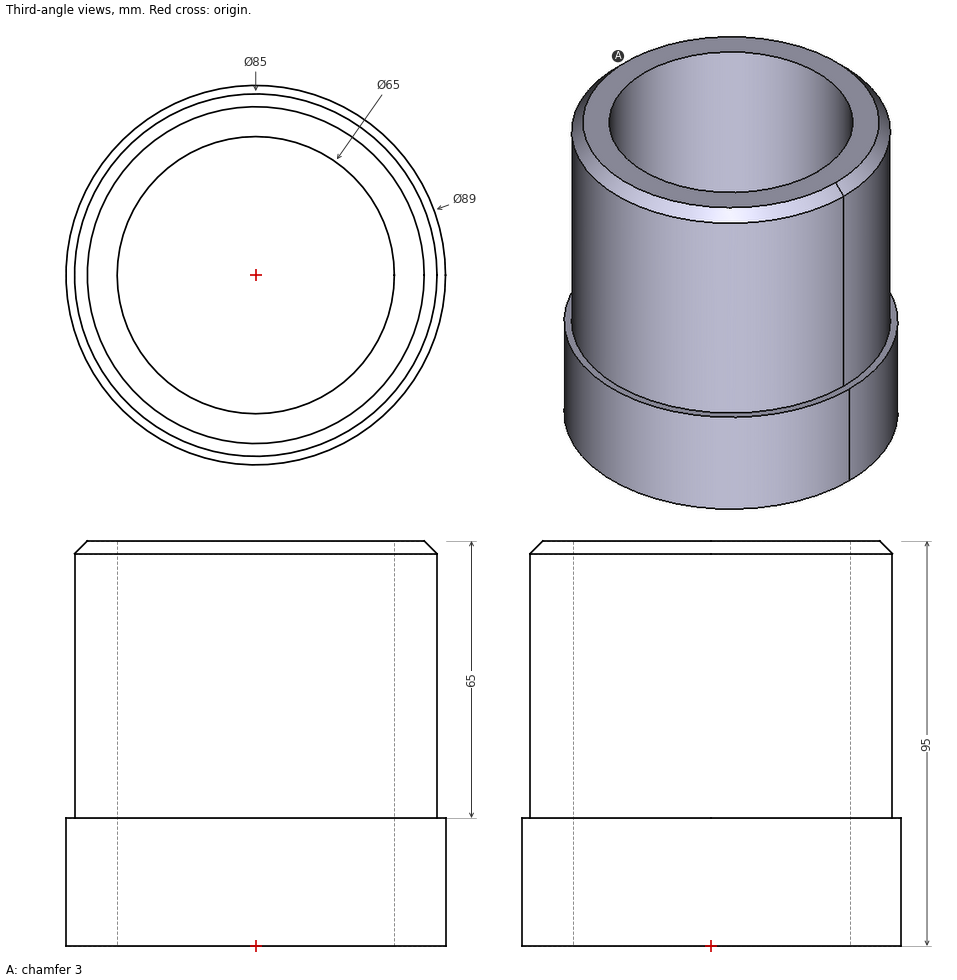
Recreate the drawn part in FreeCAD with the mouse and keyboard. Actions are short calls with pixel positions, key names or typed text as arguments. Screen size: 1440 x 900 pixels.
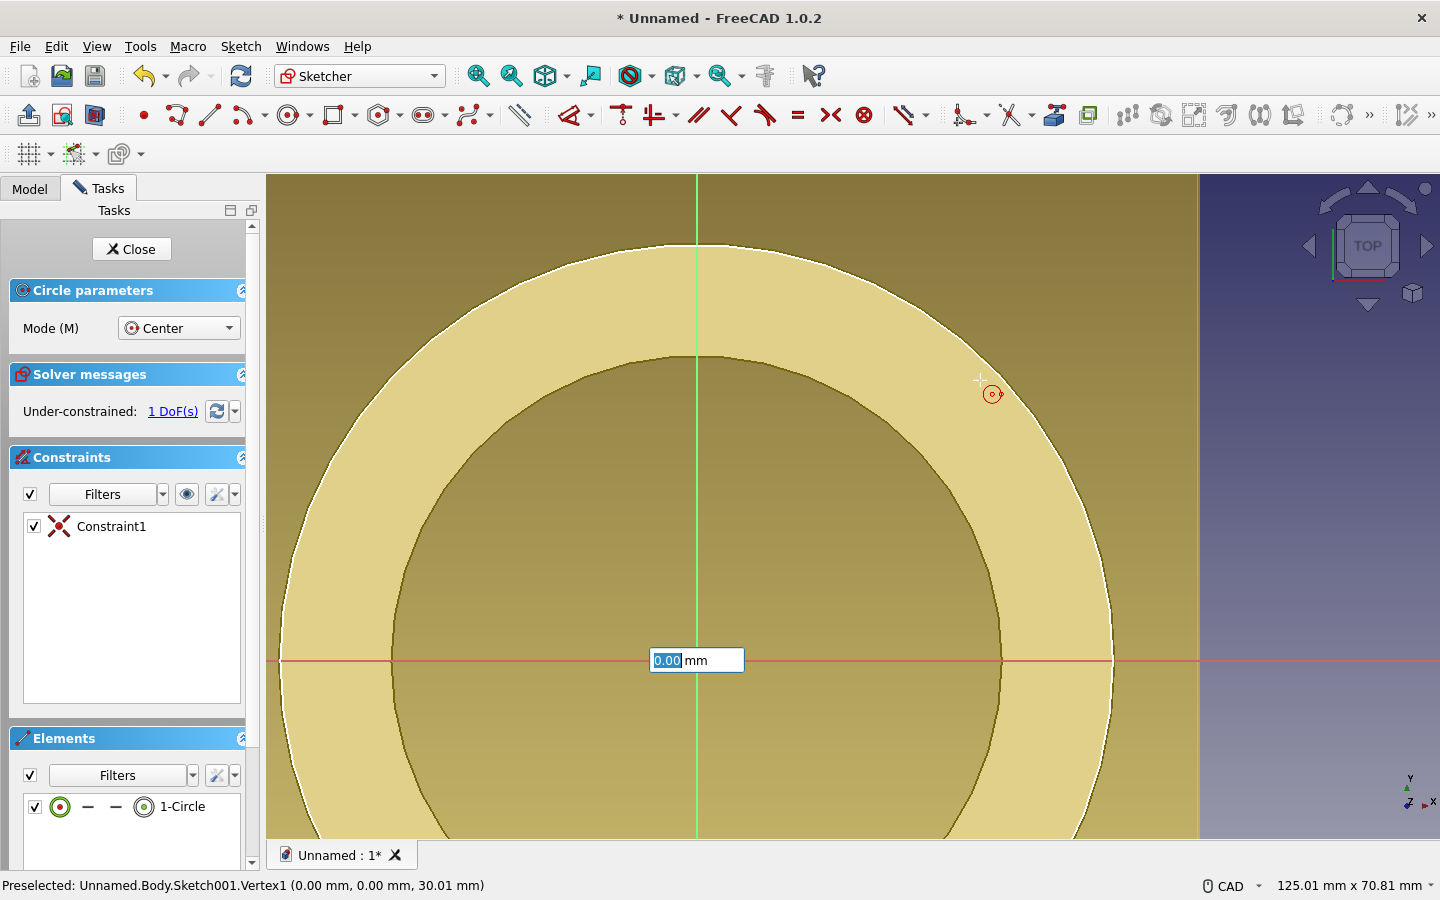
click(979, 379)
key(Escape)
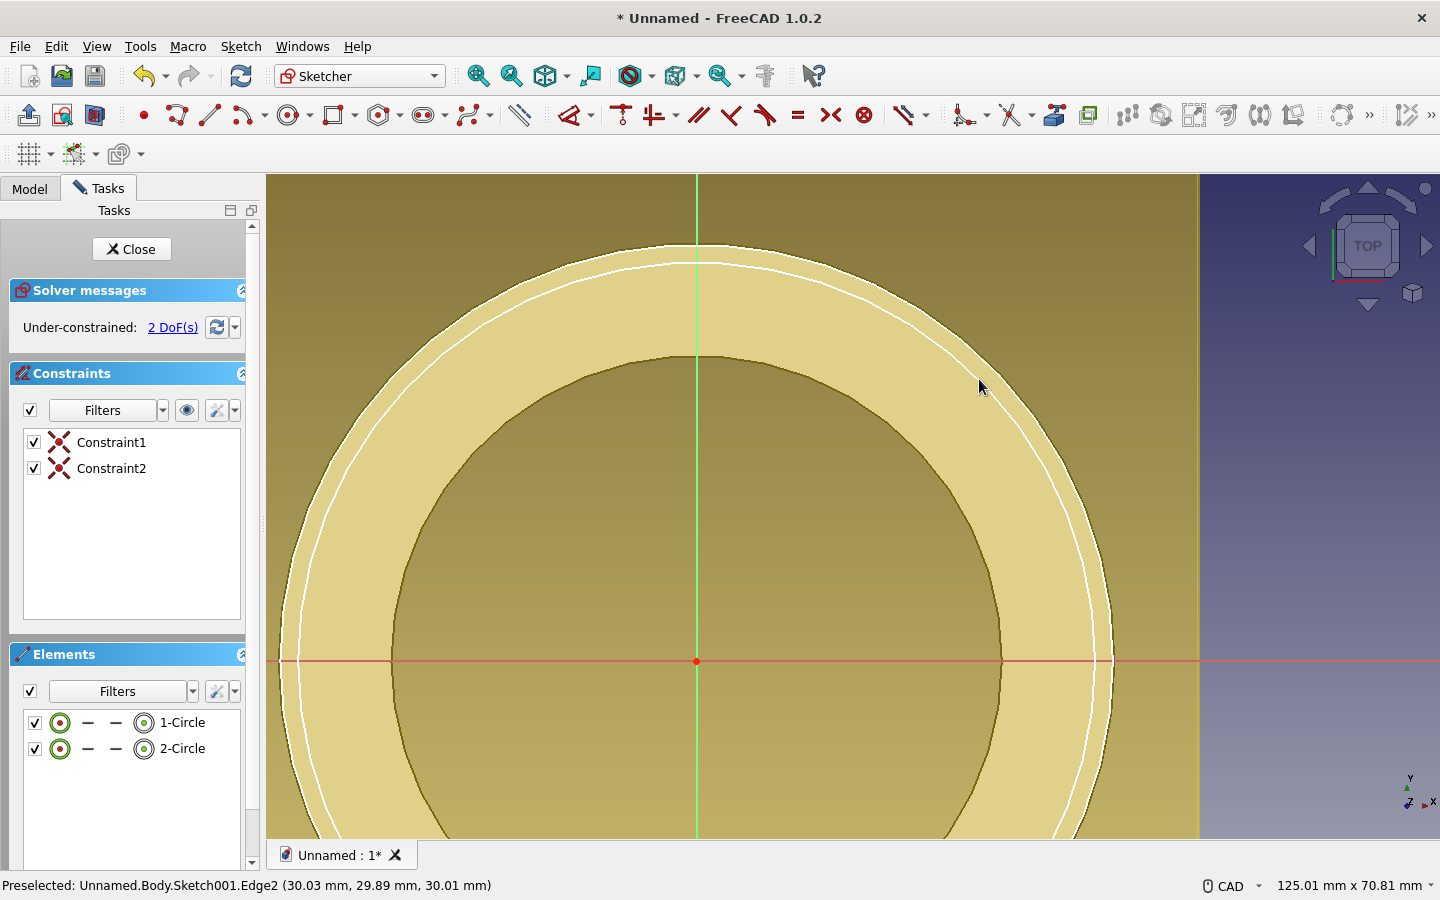
key(d)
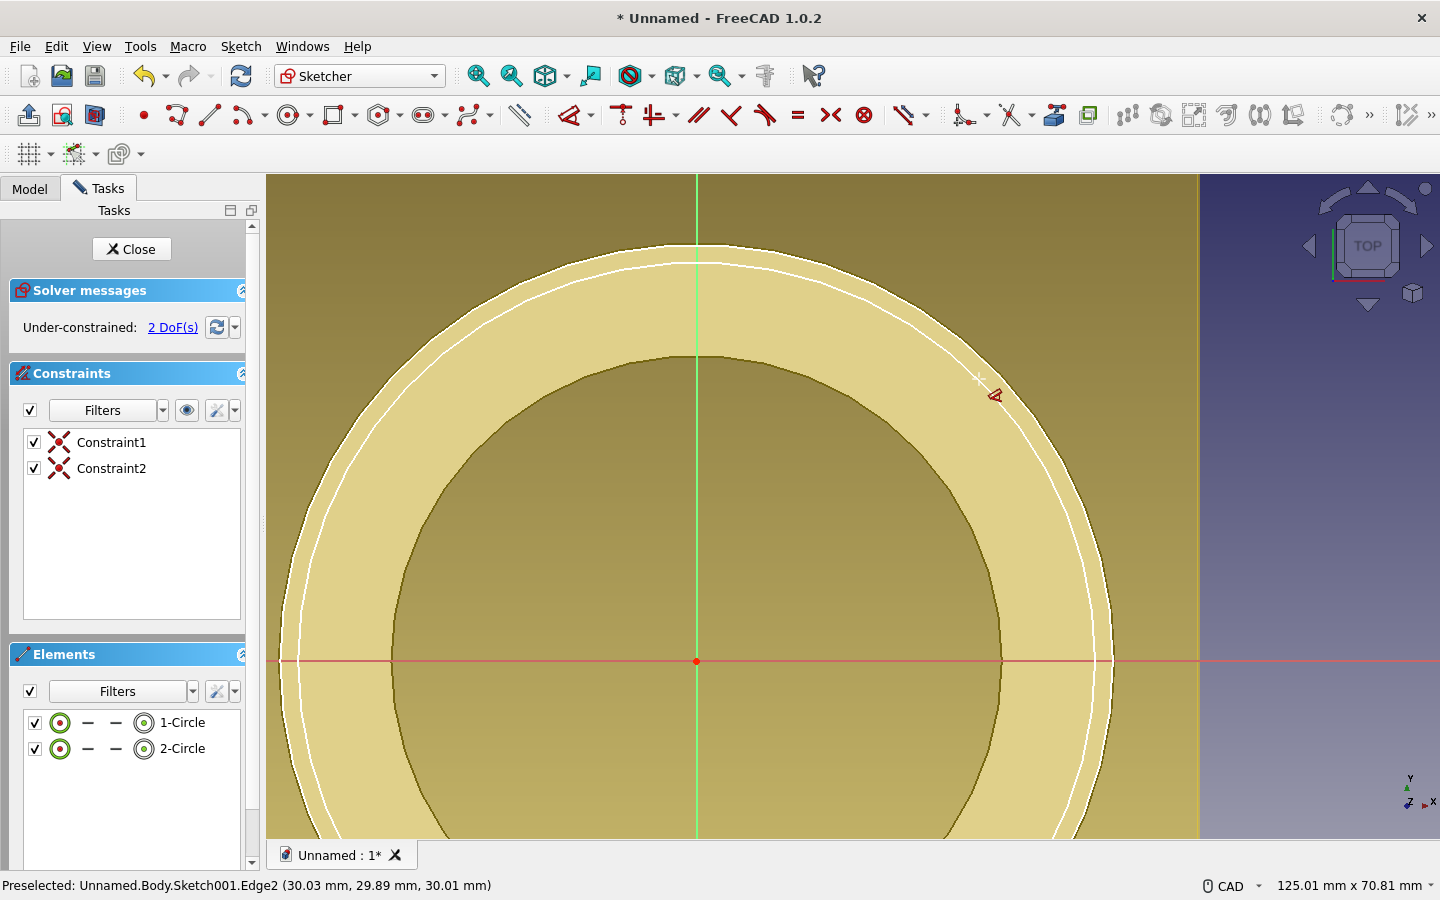
click(990, 366)
click(1013, 343)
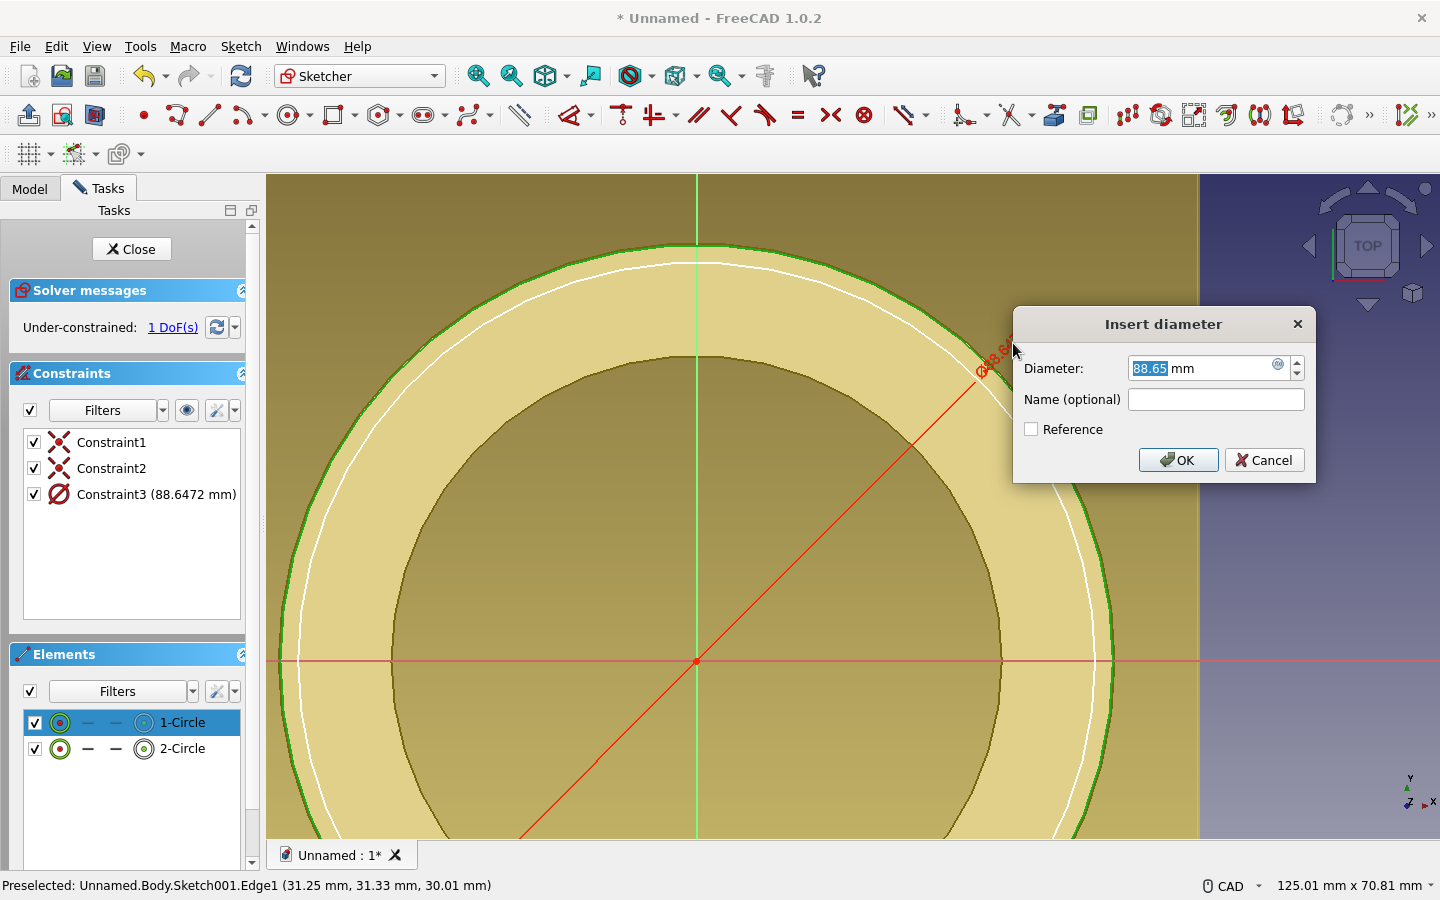
text(89)
key(Return)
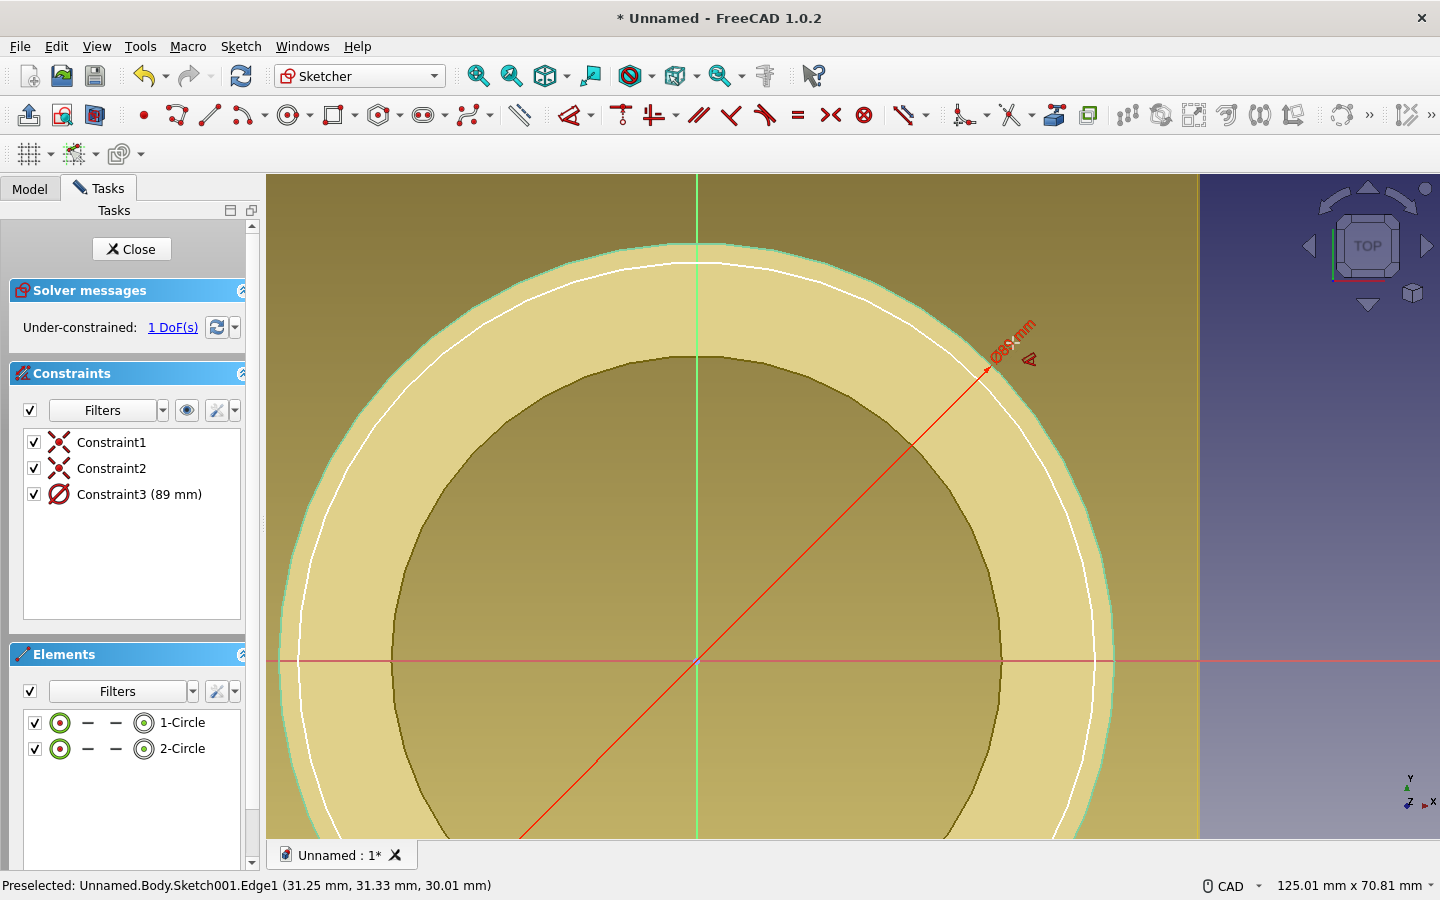
click(978, 379)
click(1132, 533)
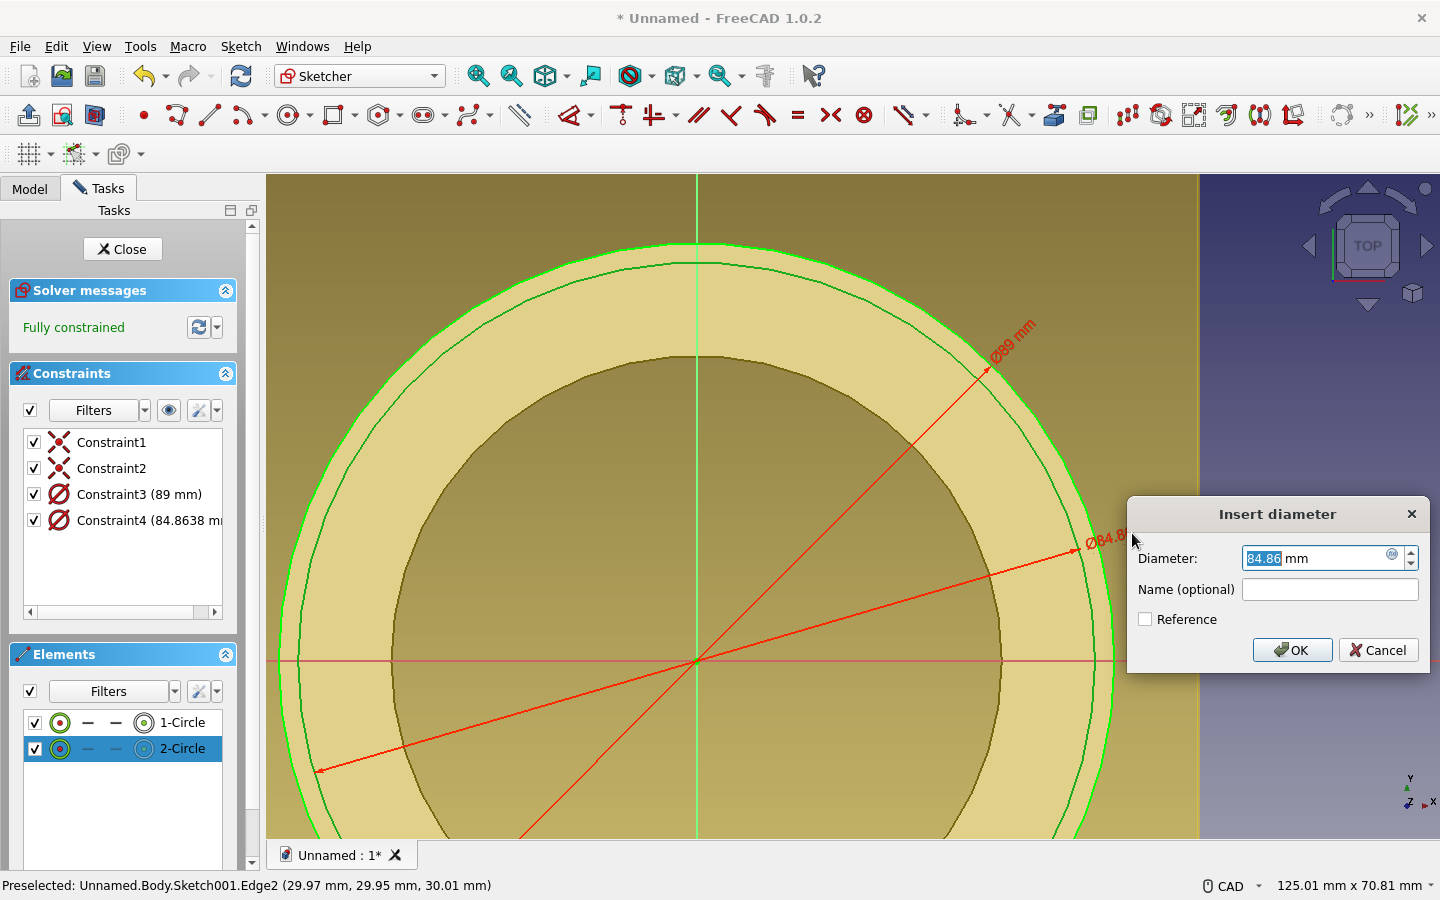
text(85)
key(Return)
key(Escape)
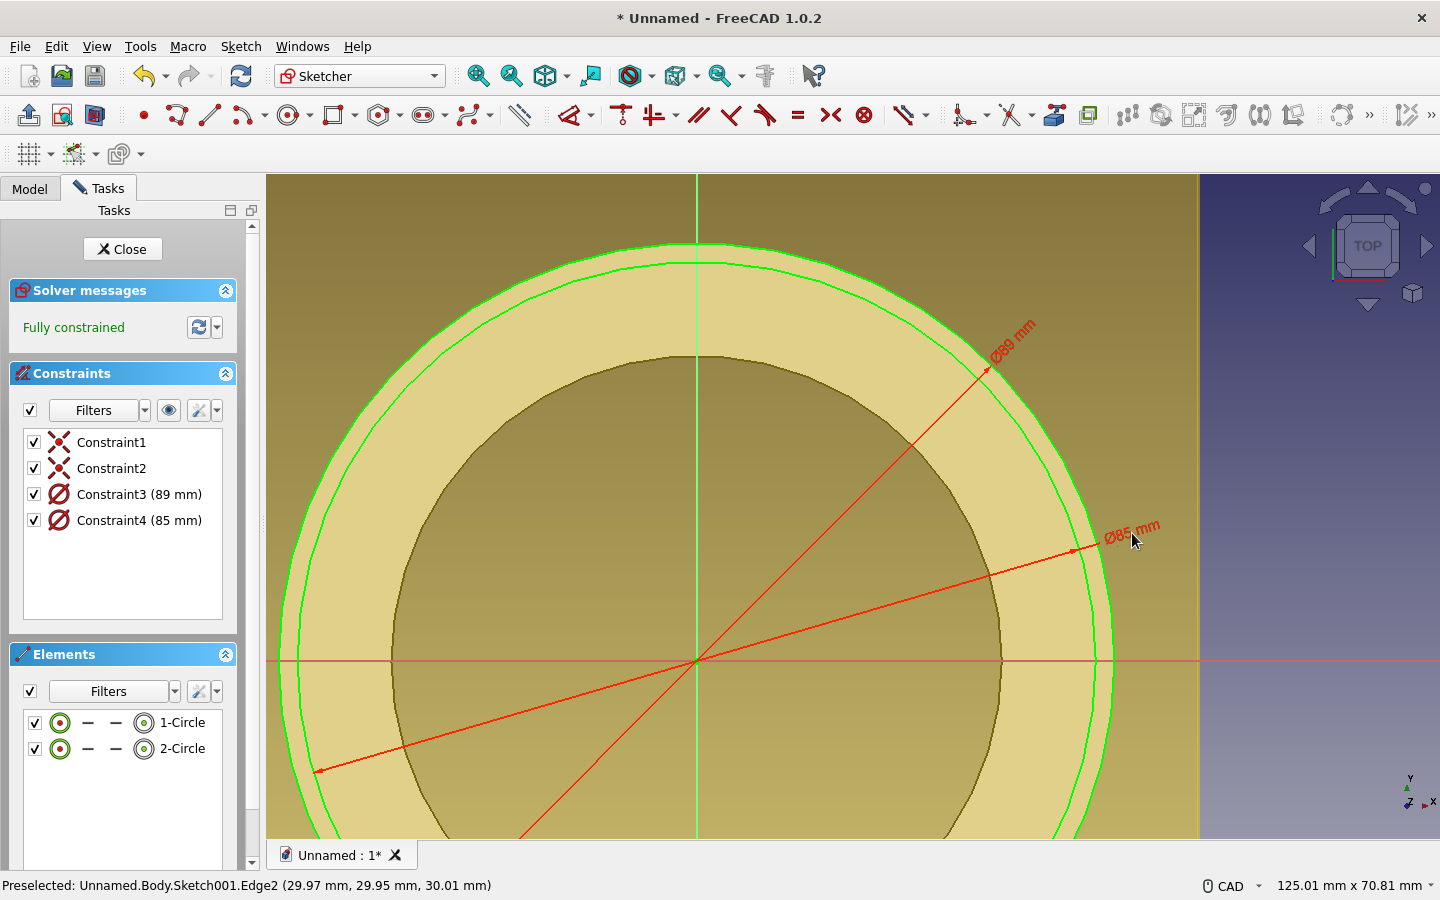
click(123, 249)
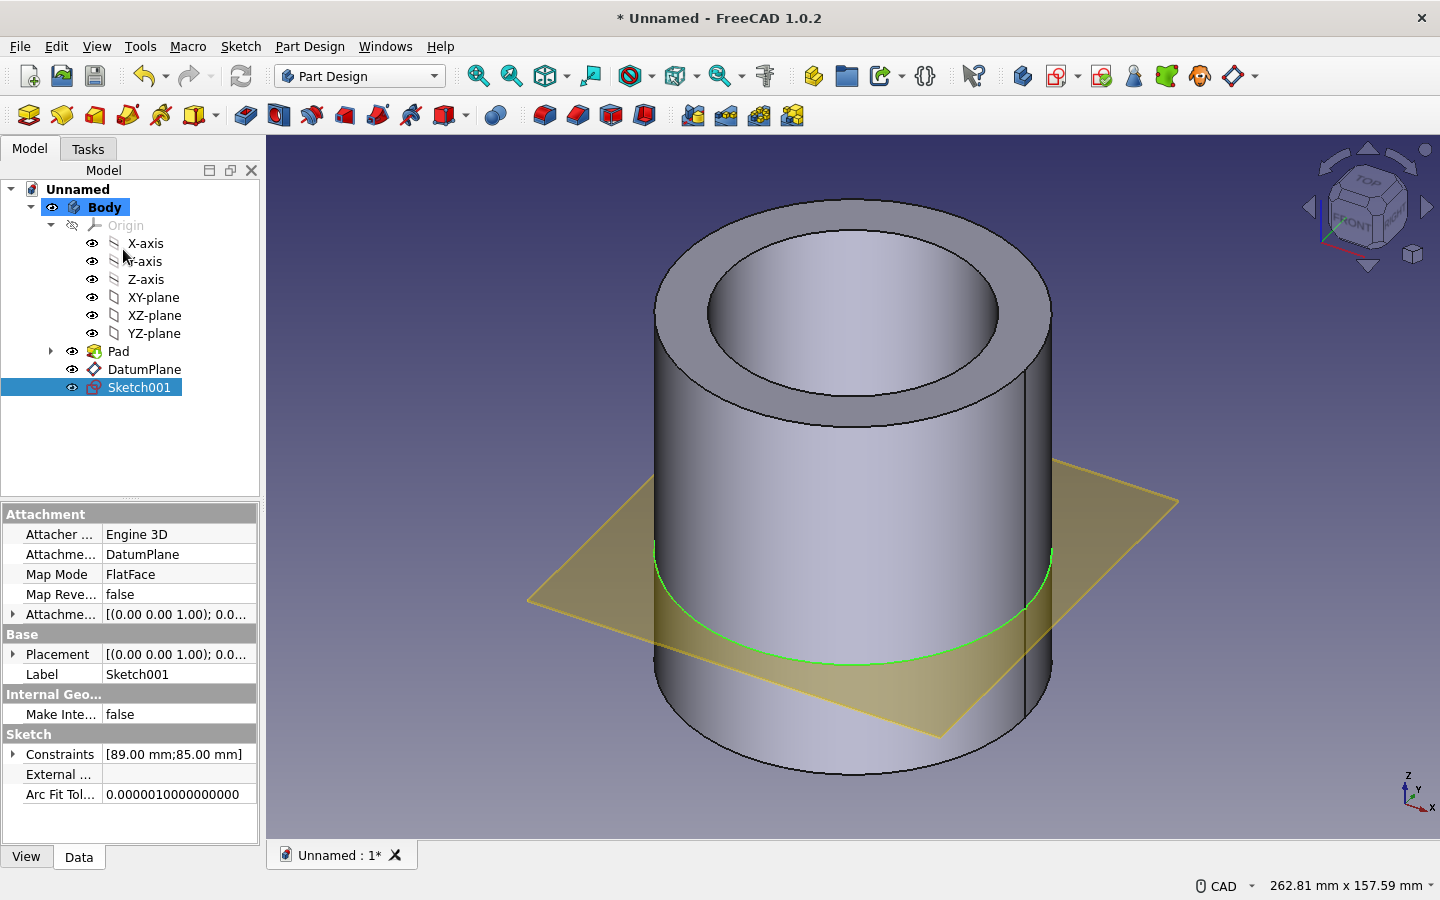
click(246, 116)